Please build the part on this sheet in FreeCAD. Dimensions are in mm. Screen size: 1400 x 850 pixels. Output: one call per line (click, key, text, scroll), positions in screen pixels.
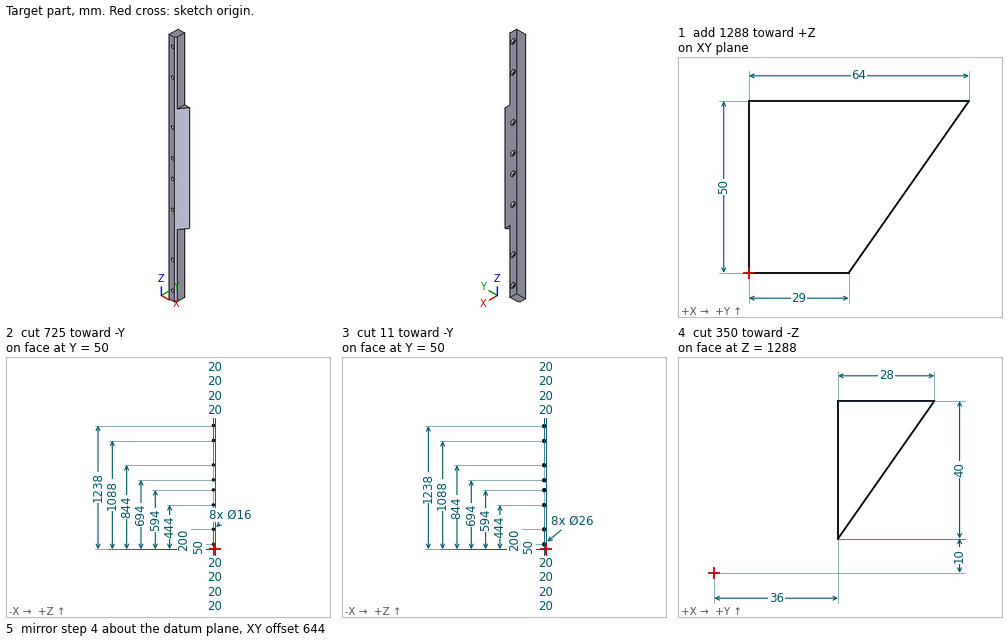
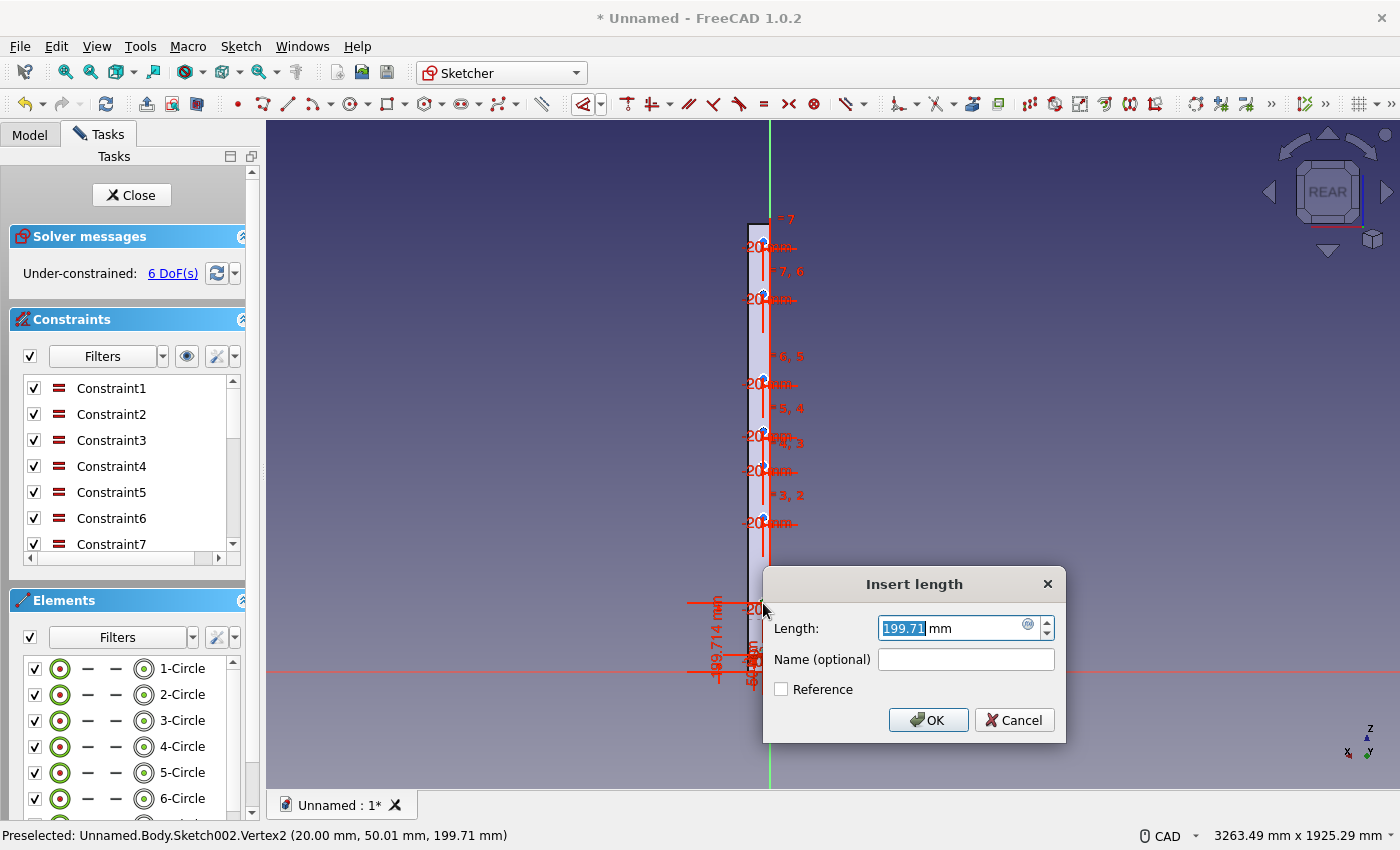
text(200)
key(Return)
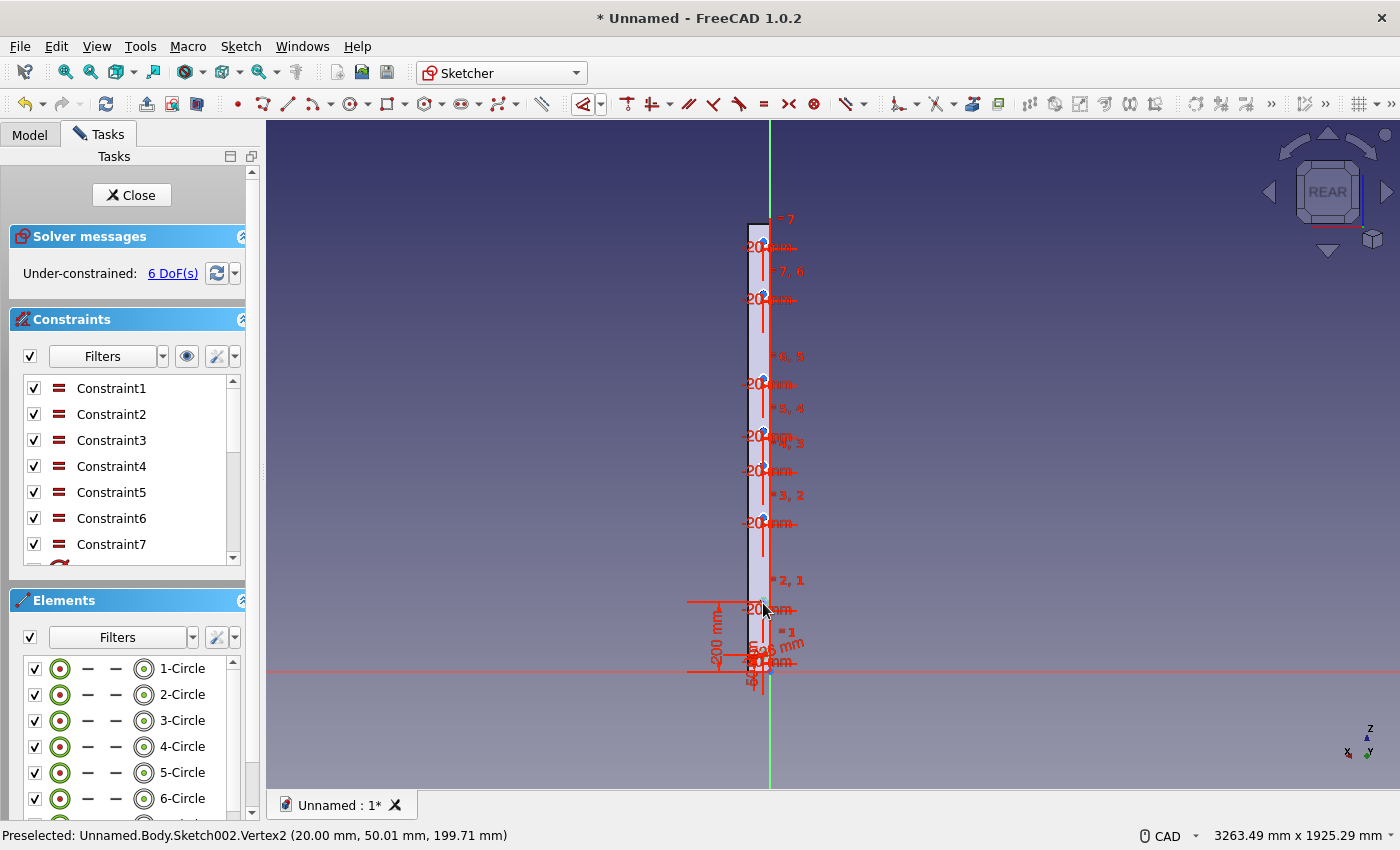
click(763, 518)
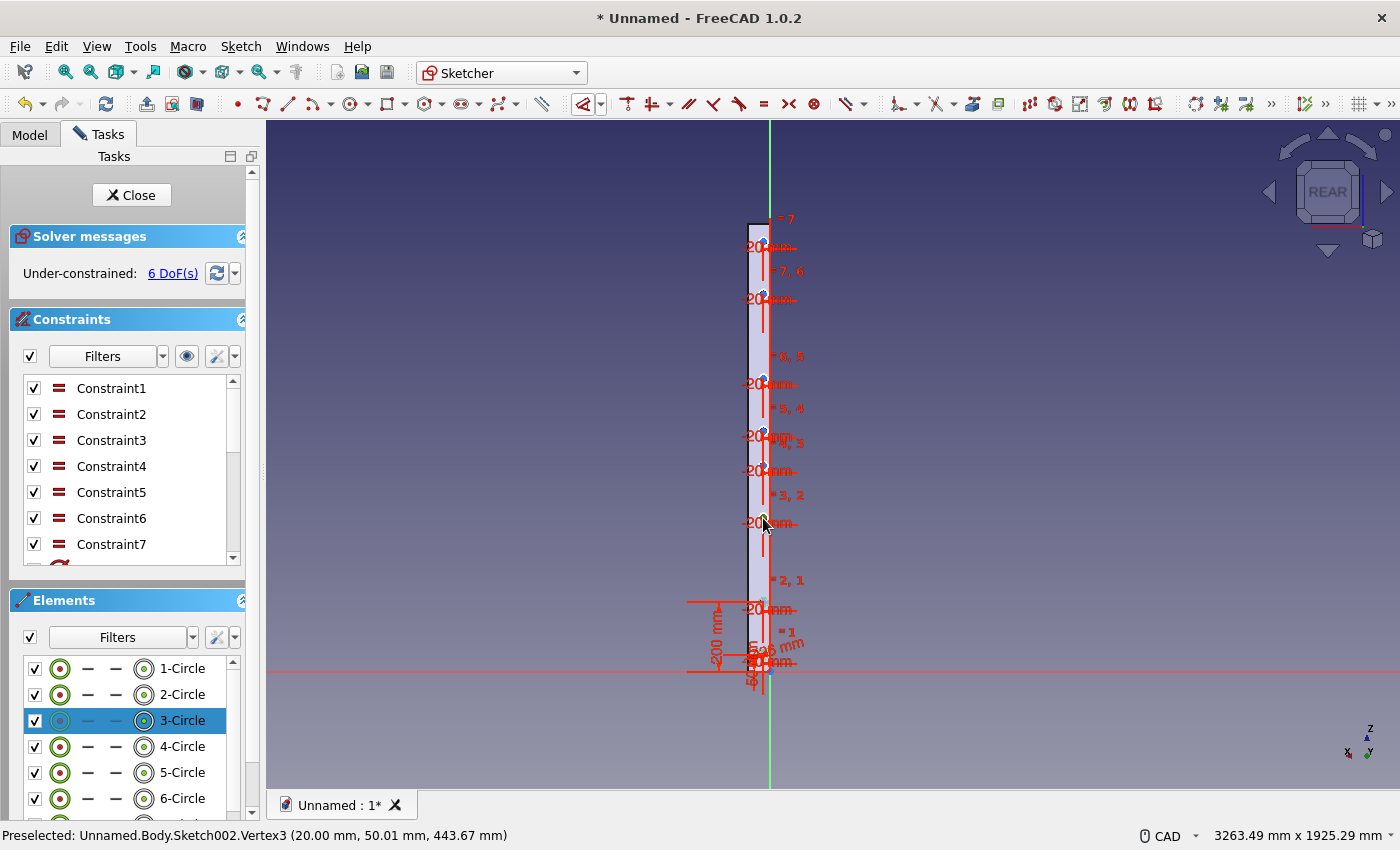
click(600, 104)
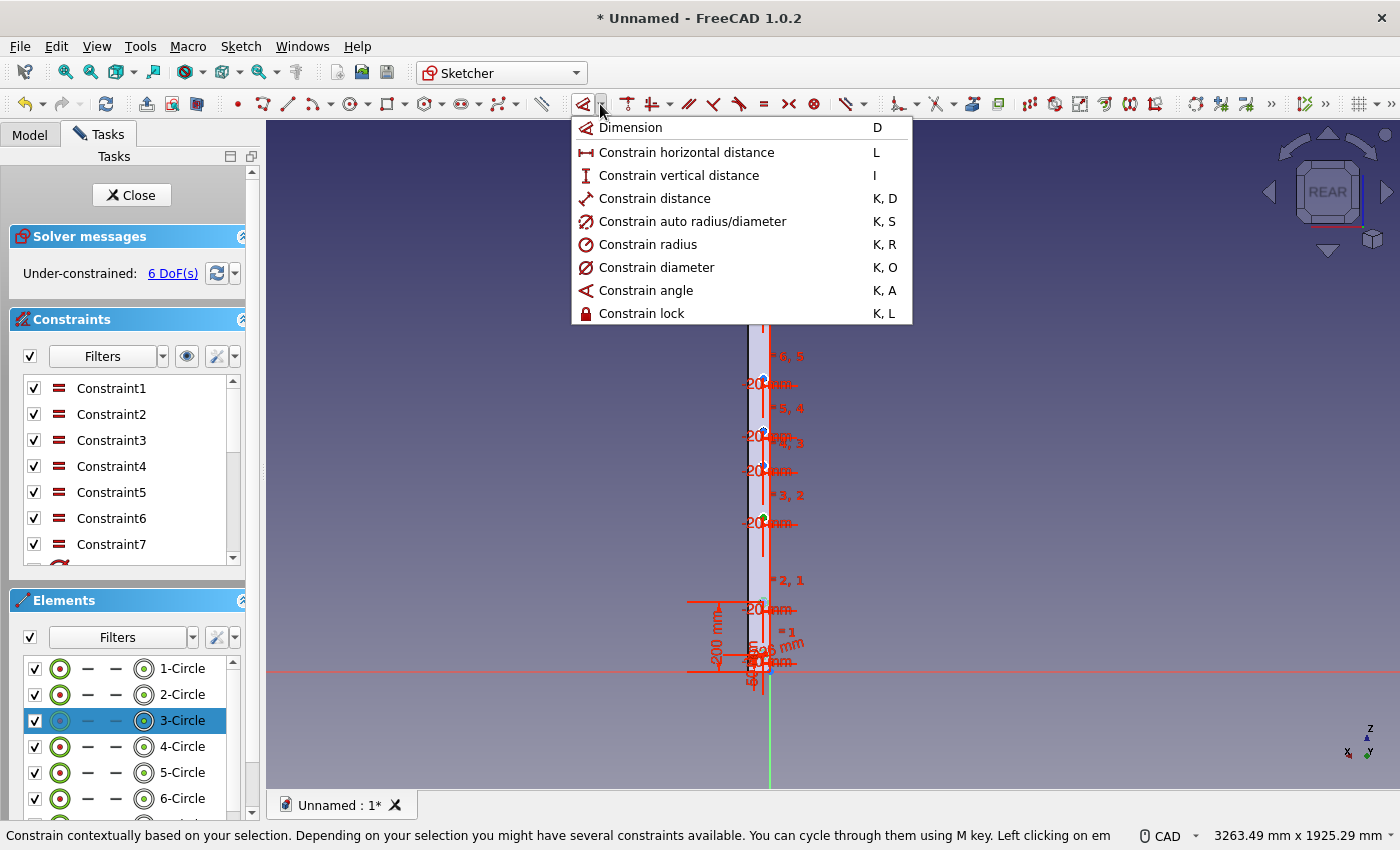
click(742, 176)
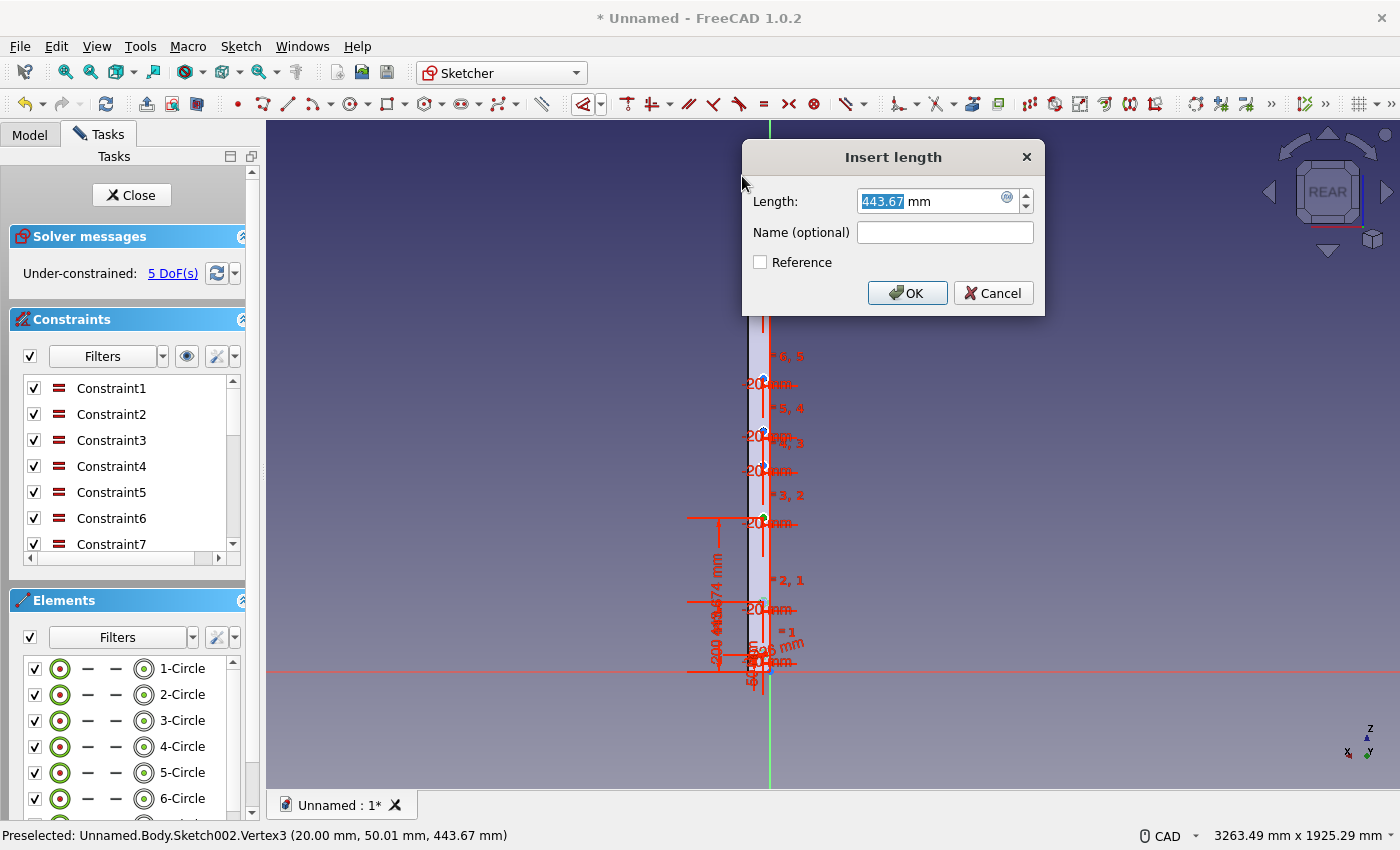
text(444)
key(Return)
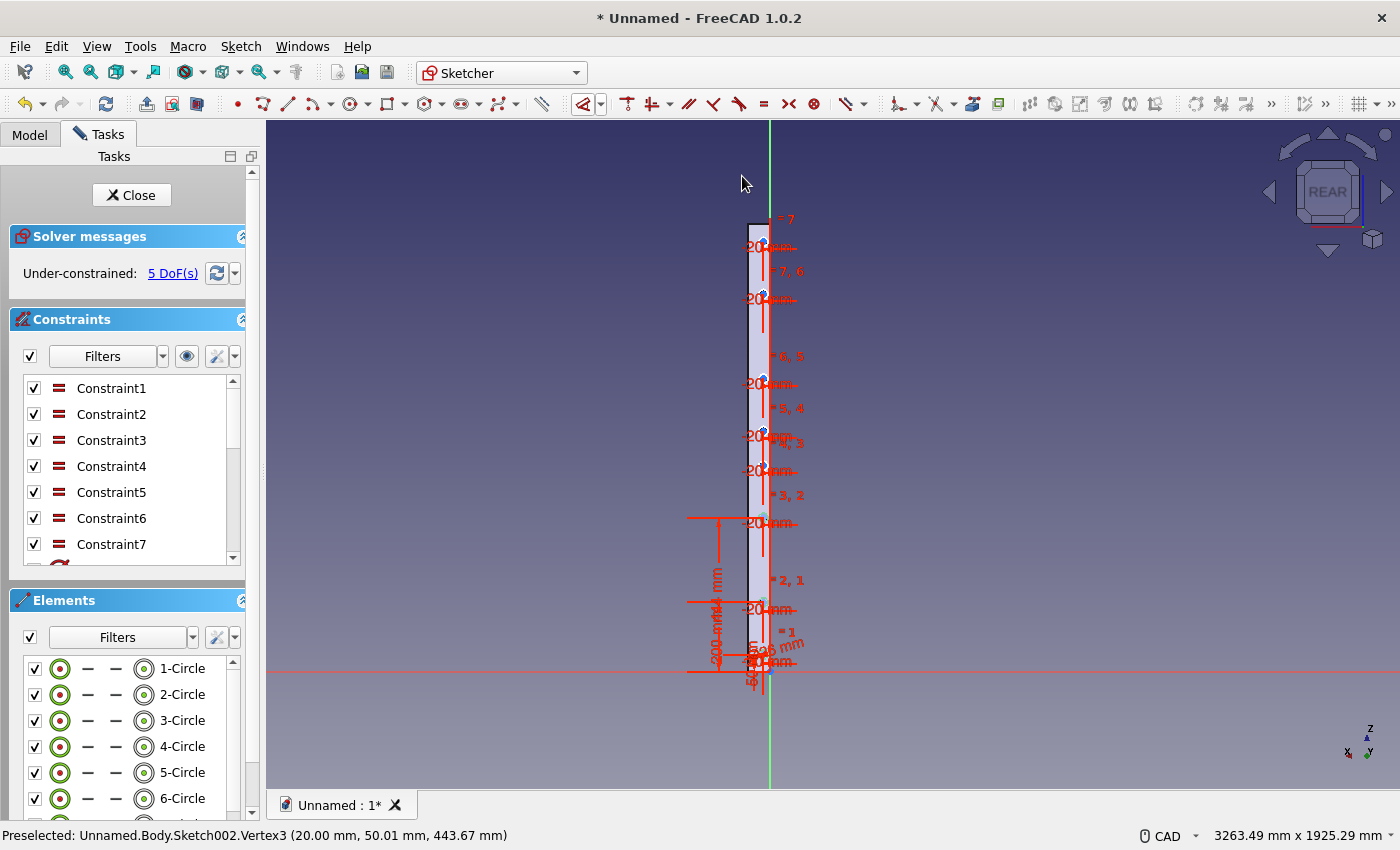
click(763, 466)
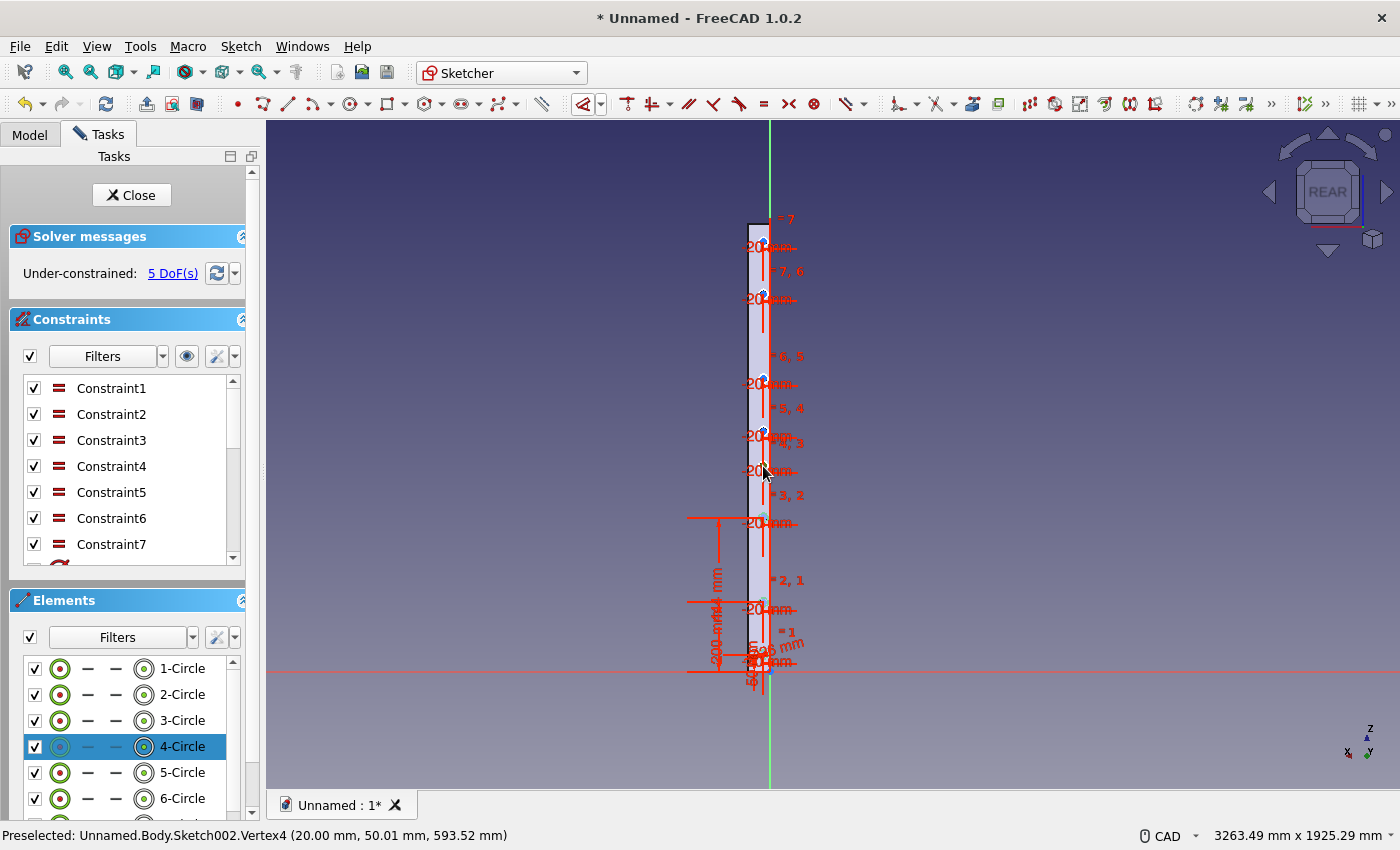
key(i)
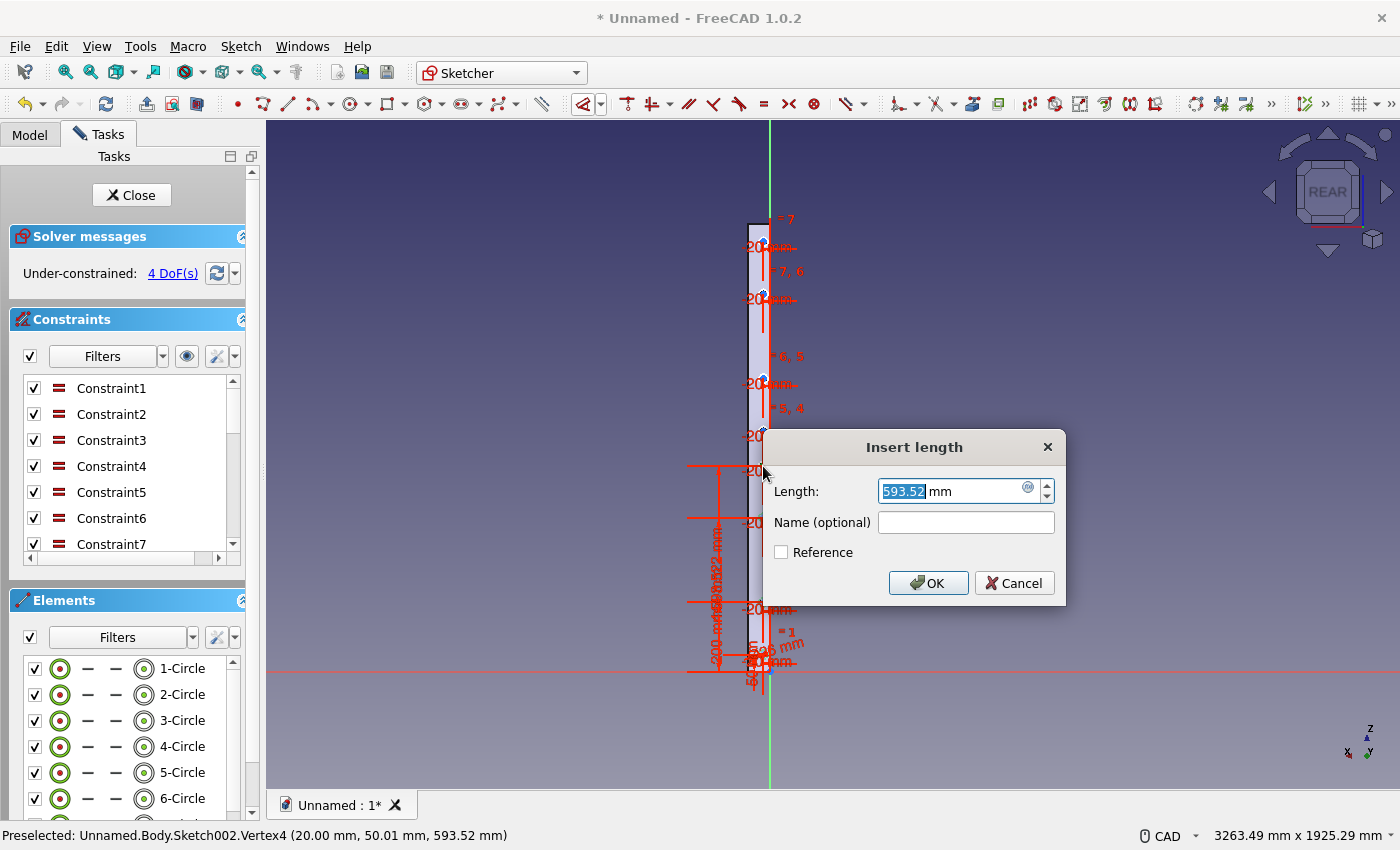
text(594)
key(Return)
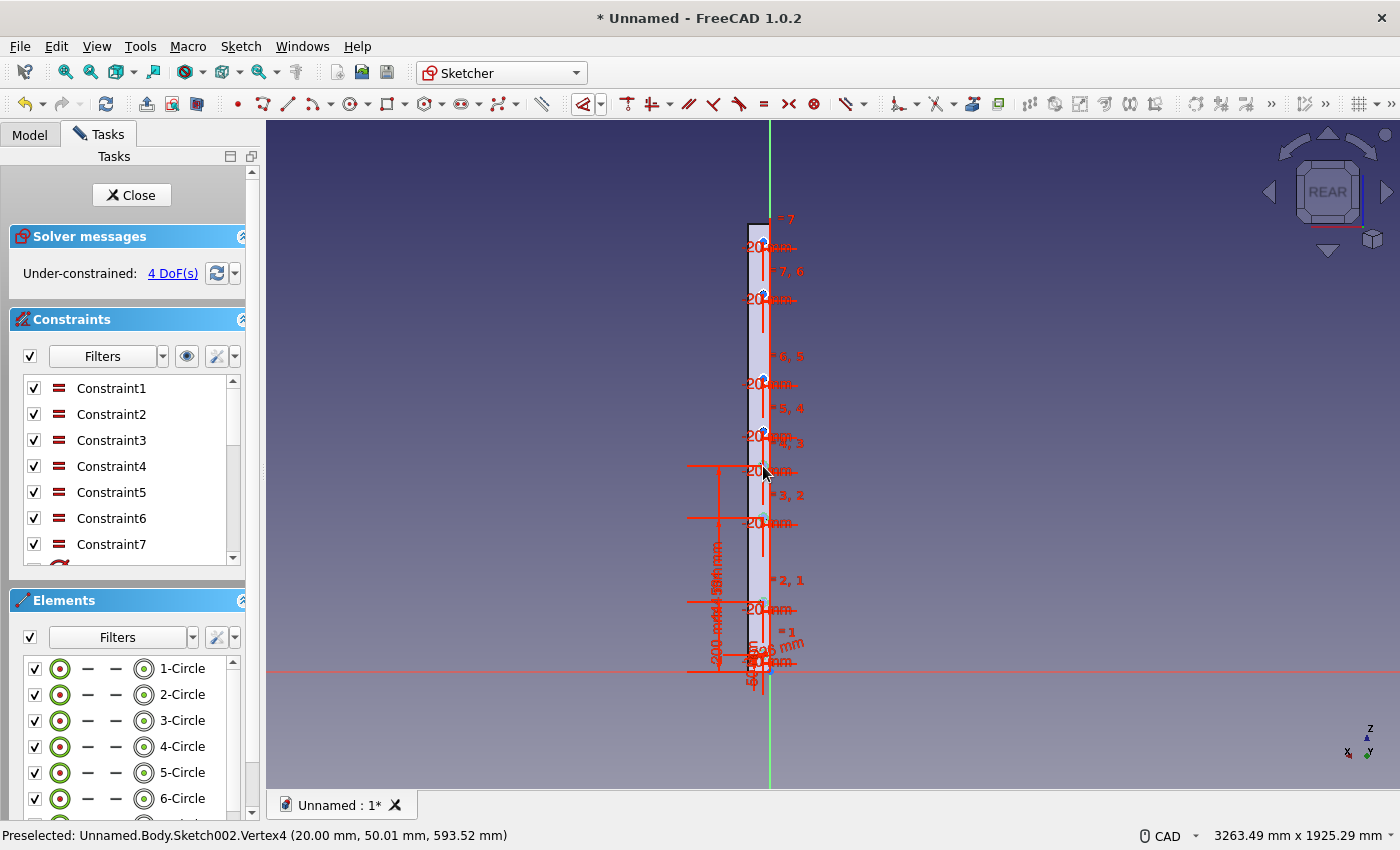
click(763, 431)